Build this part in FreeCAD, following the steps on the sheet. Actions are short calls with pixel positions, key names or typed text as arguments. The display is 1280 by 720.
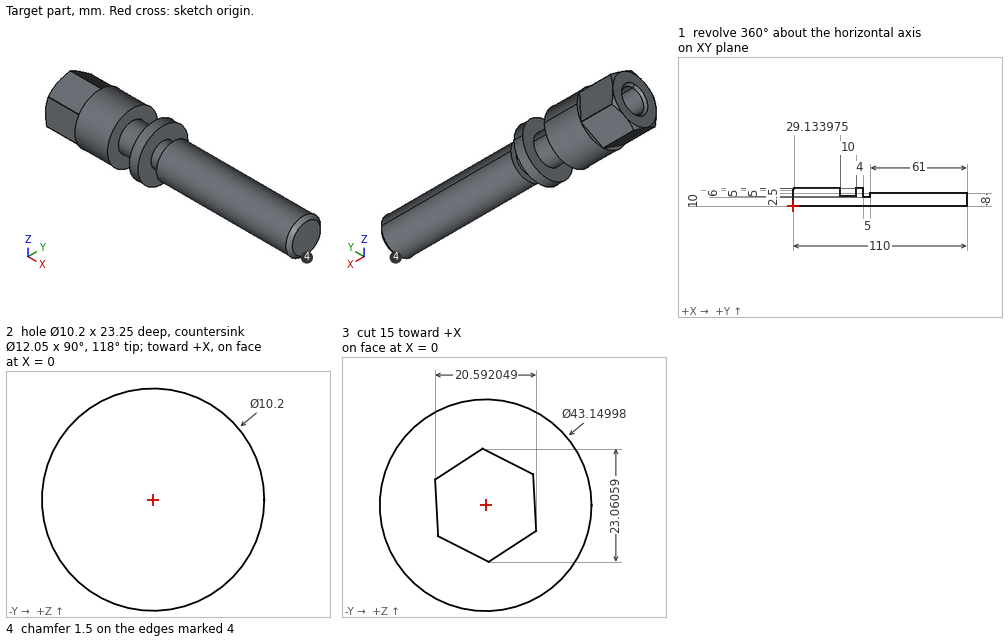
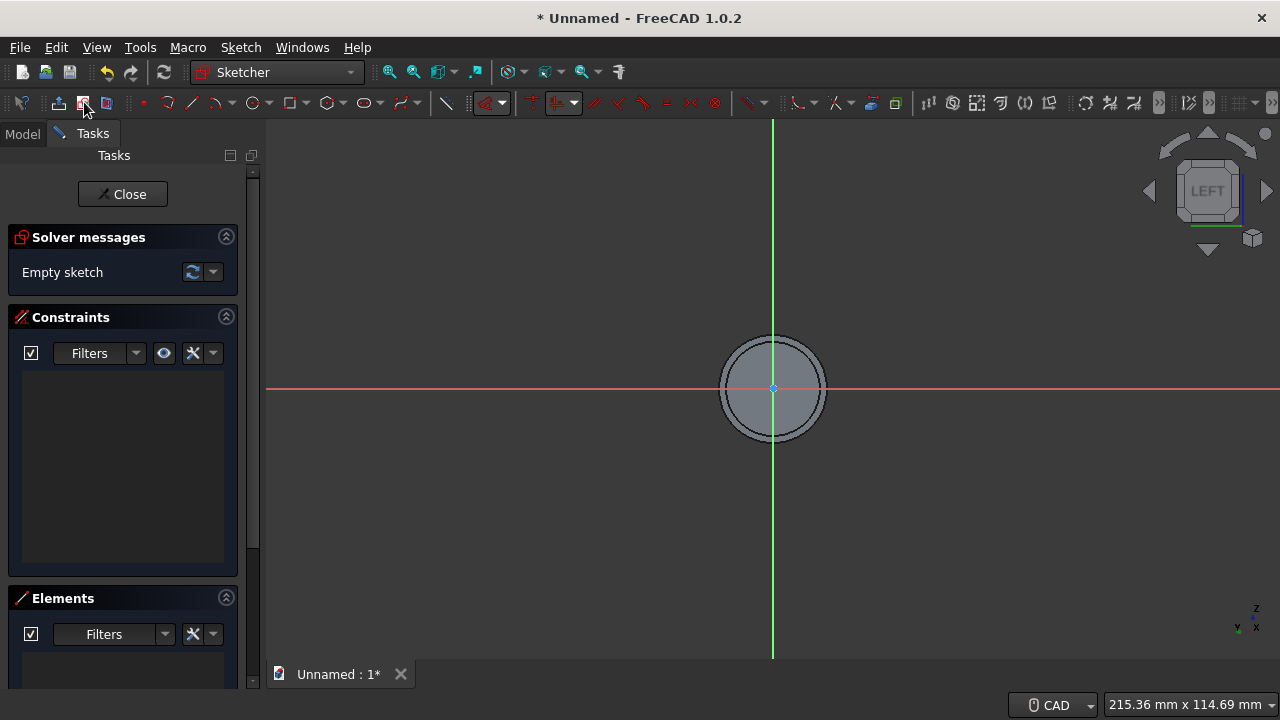
scroll(784, 389, up, 10)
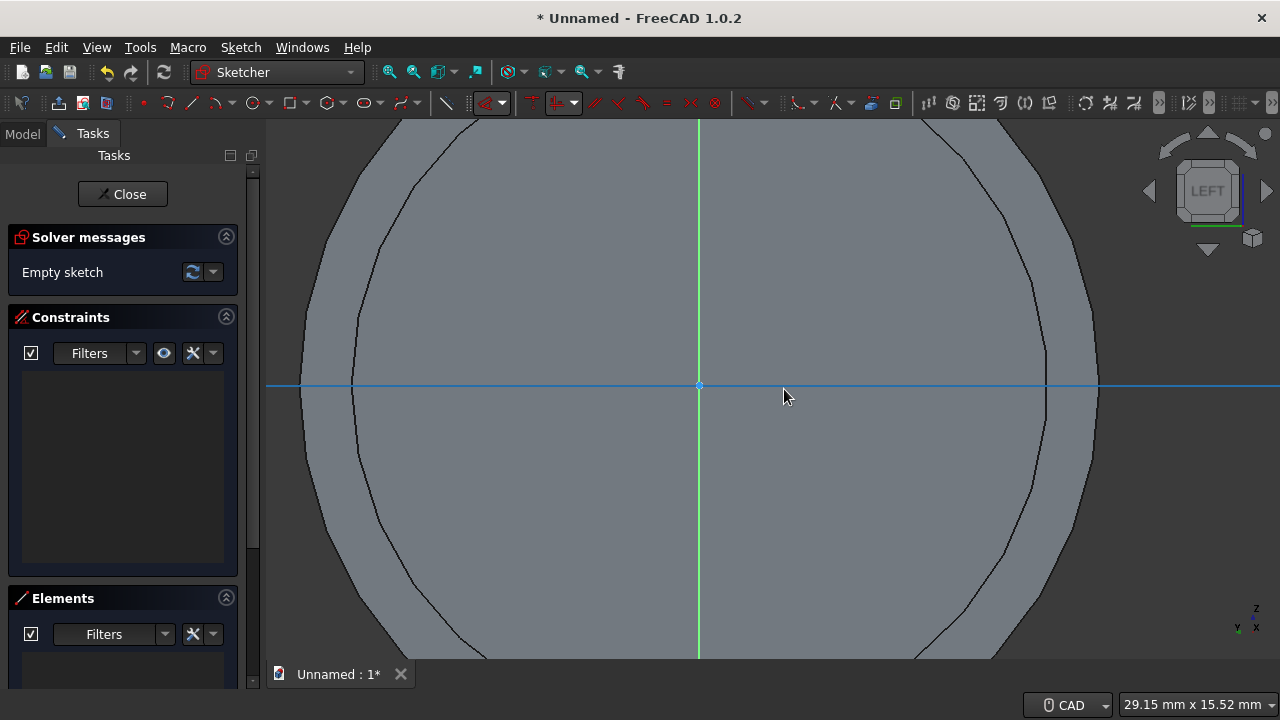
key(g)
key(c)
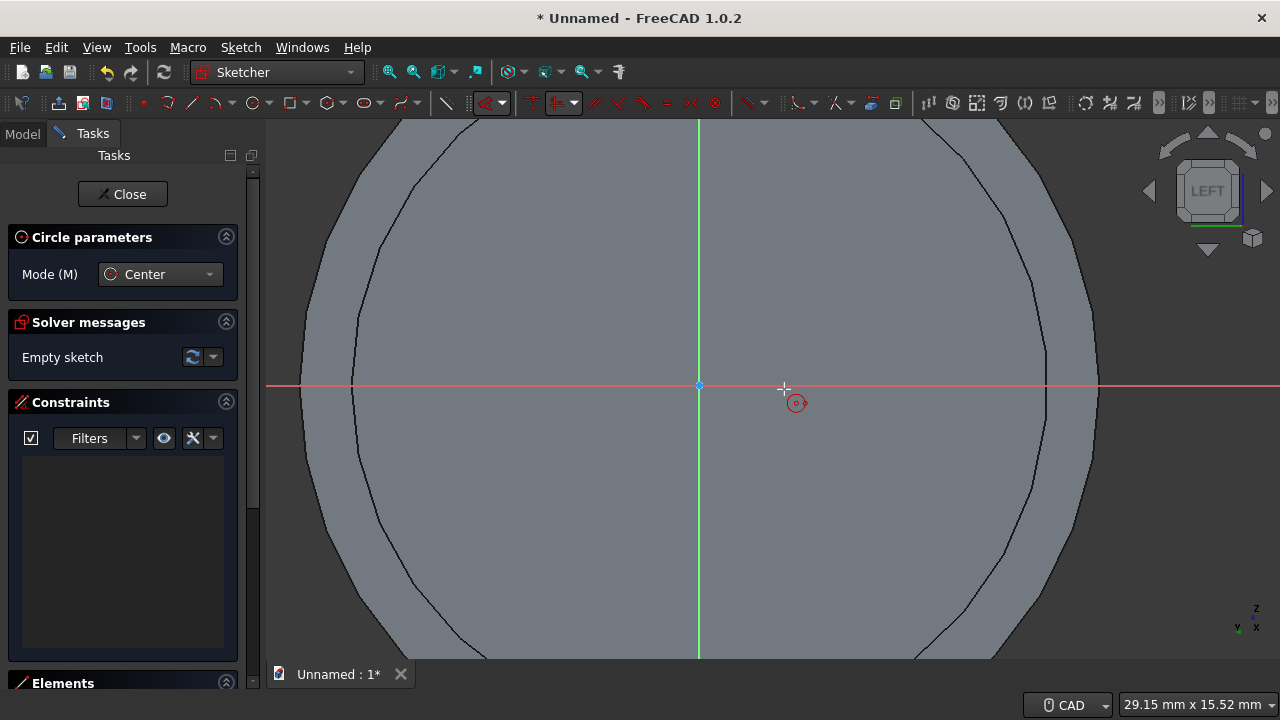
click(699, 386)
move(825, 260)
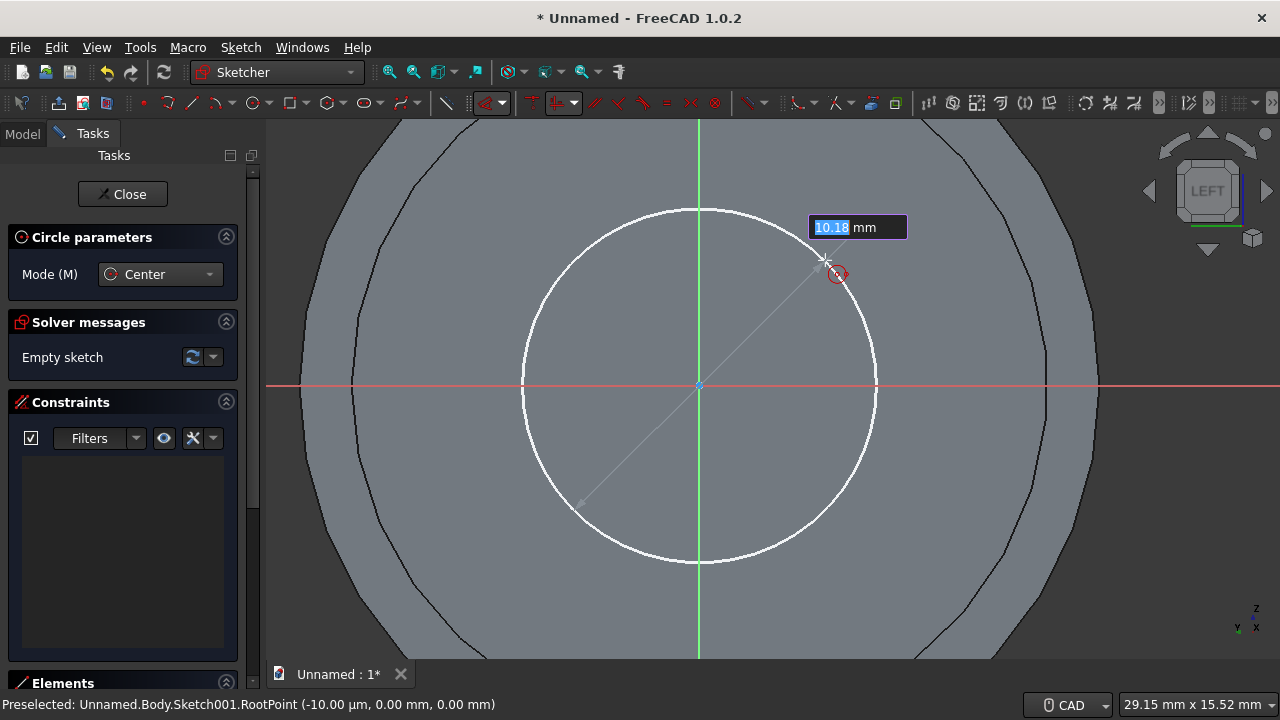
text(10.2)
key(Return)
key(Escape)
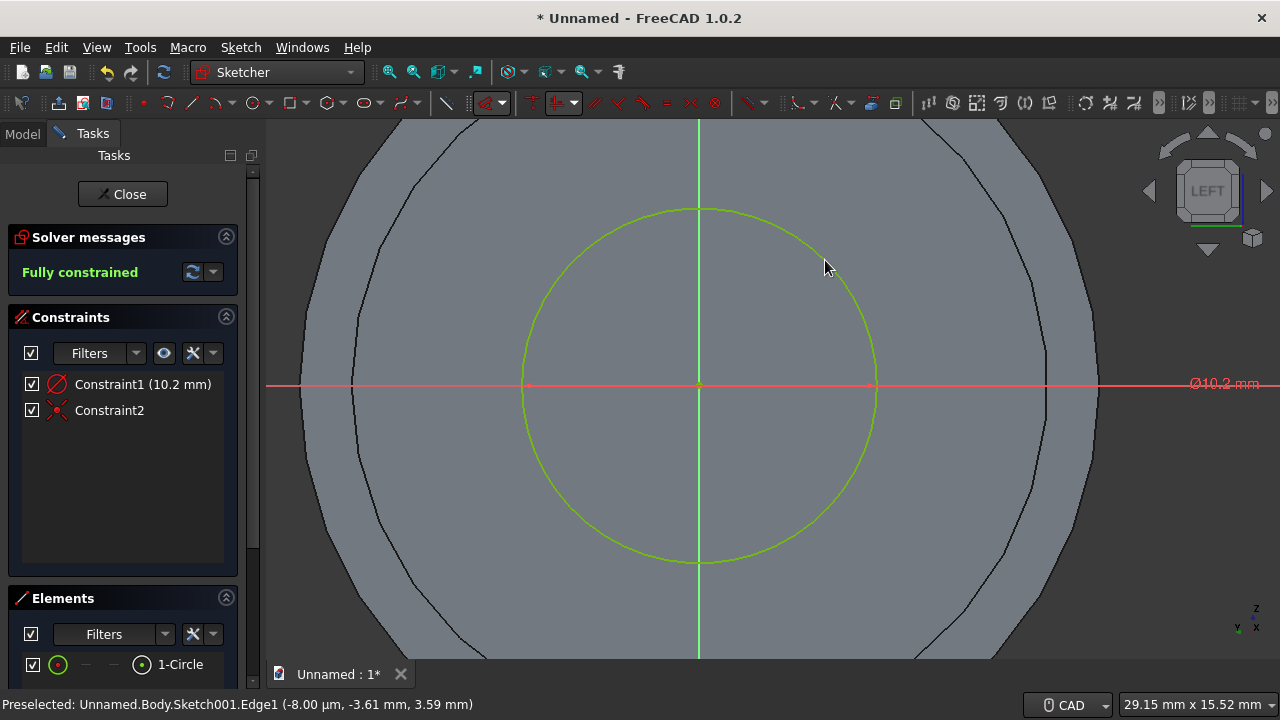
click(123, 194)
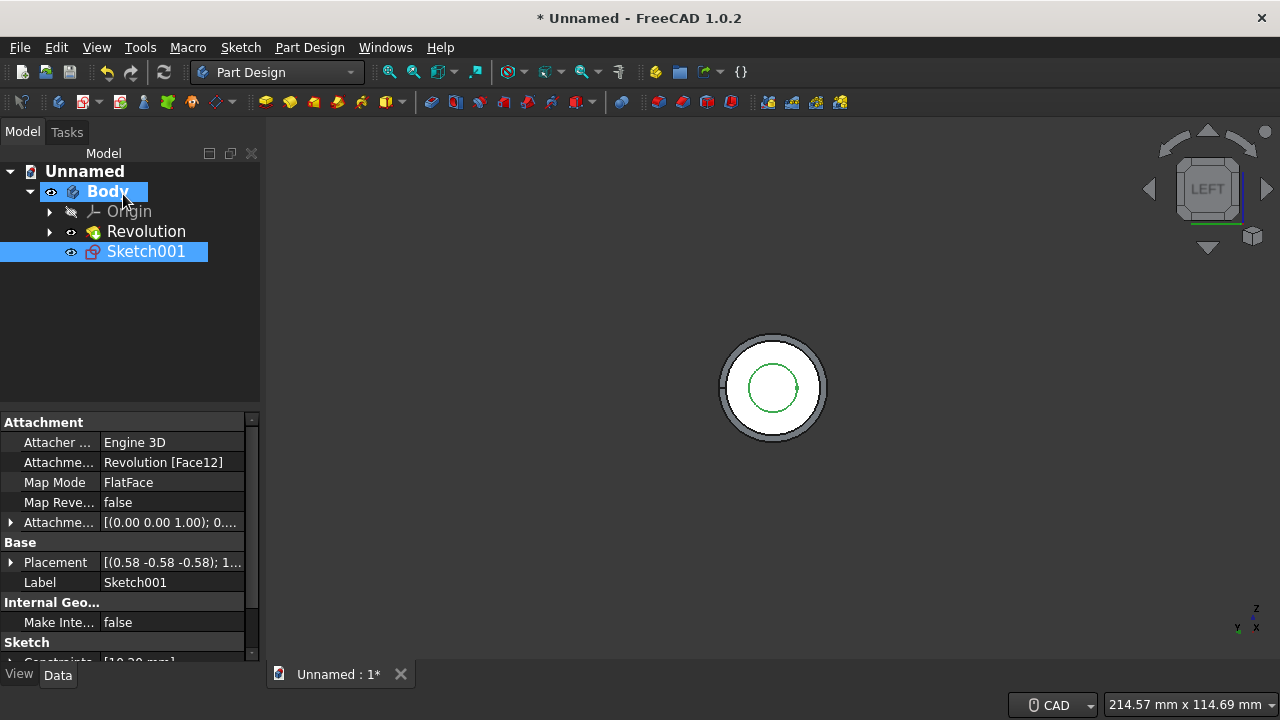
click(456, 102)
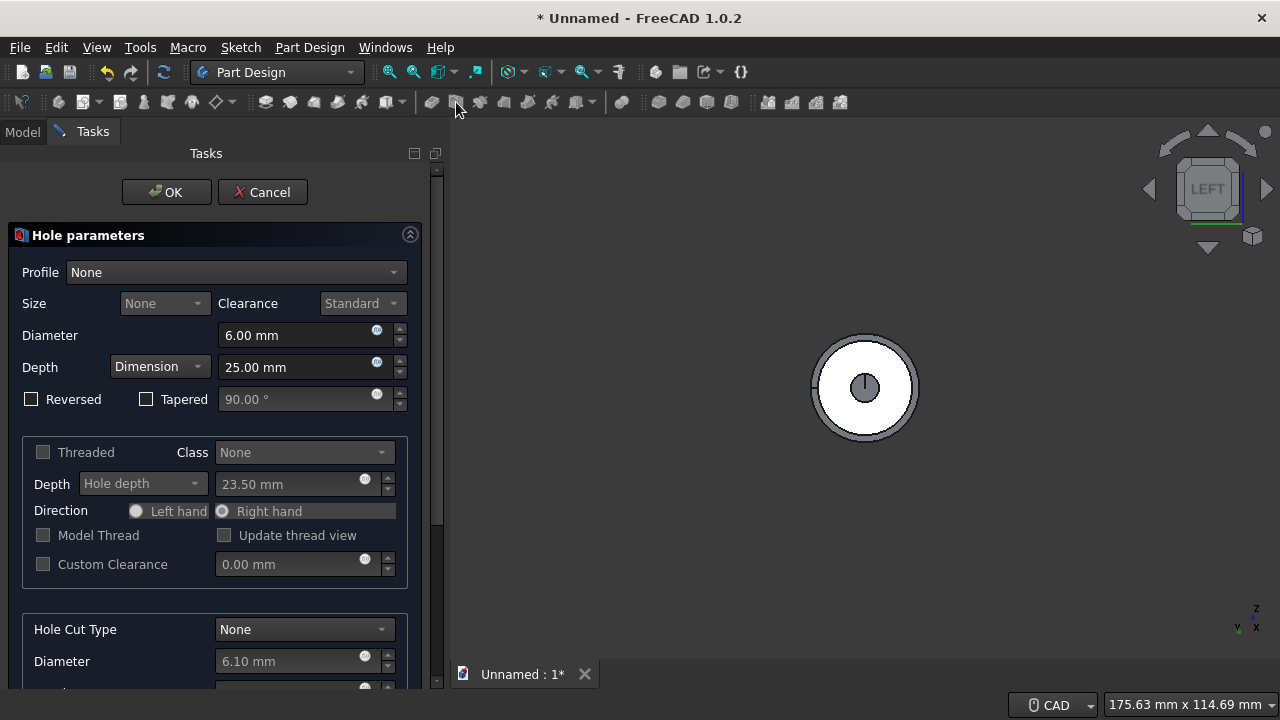
triple_click(305, 335)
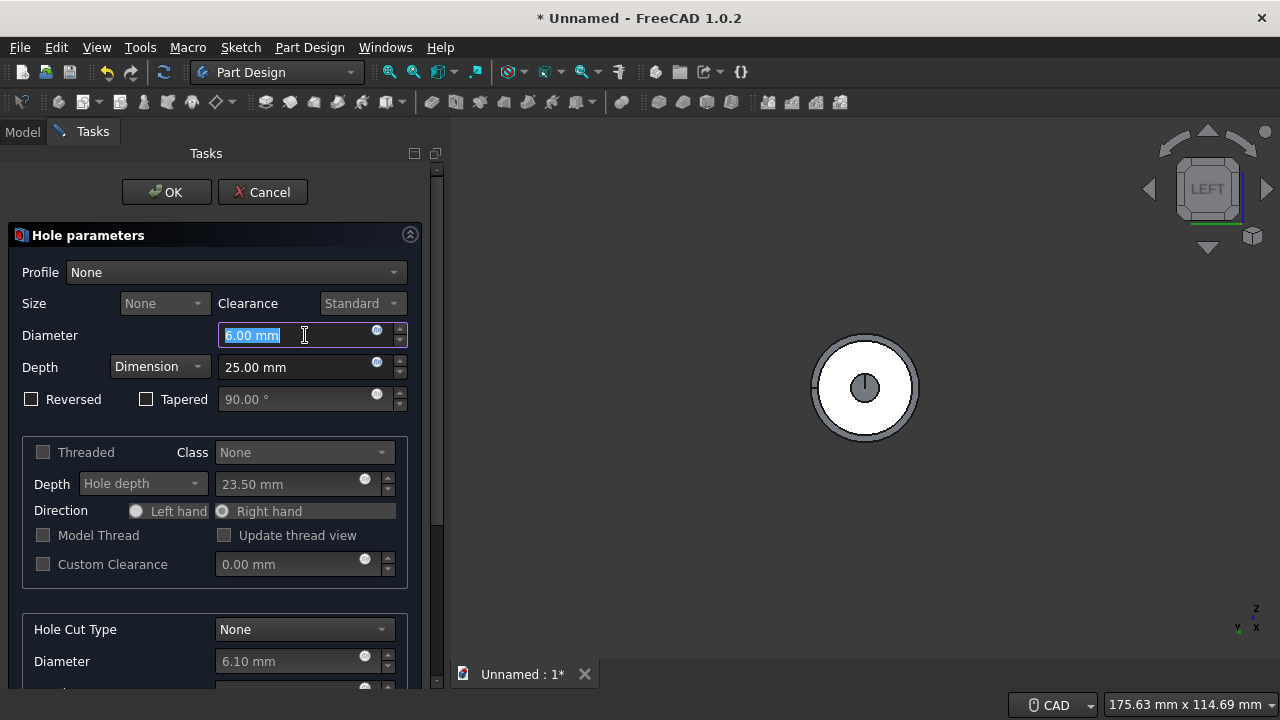
text(10.2)
key(Tab)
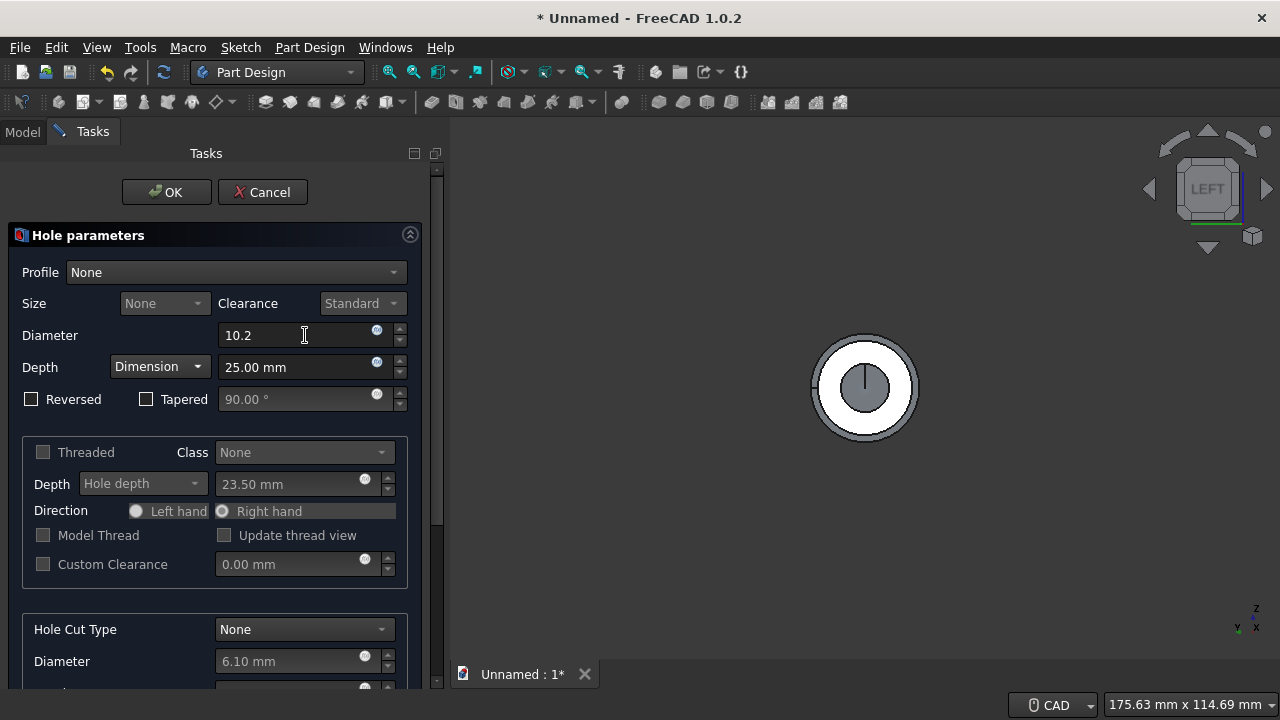
triple_click(305, 367)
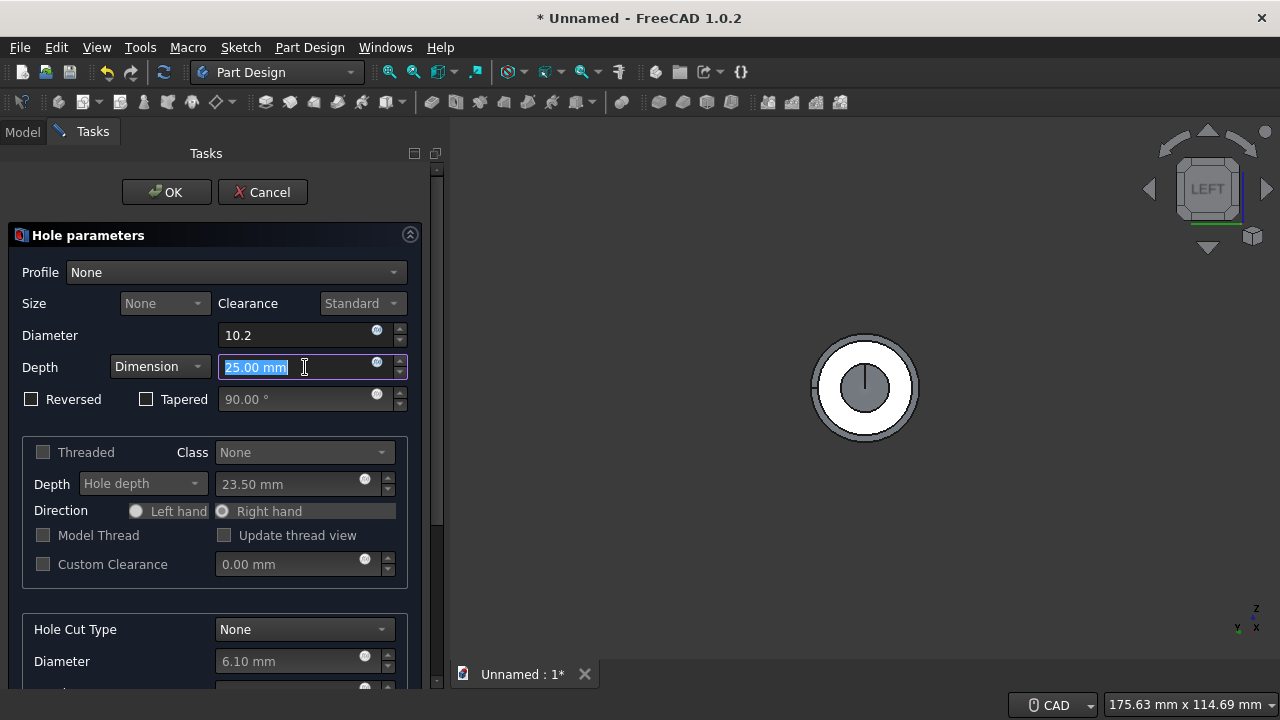
text(23.25)
key(Tab)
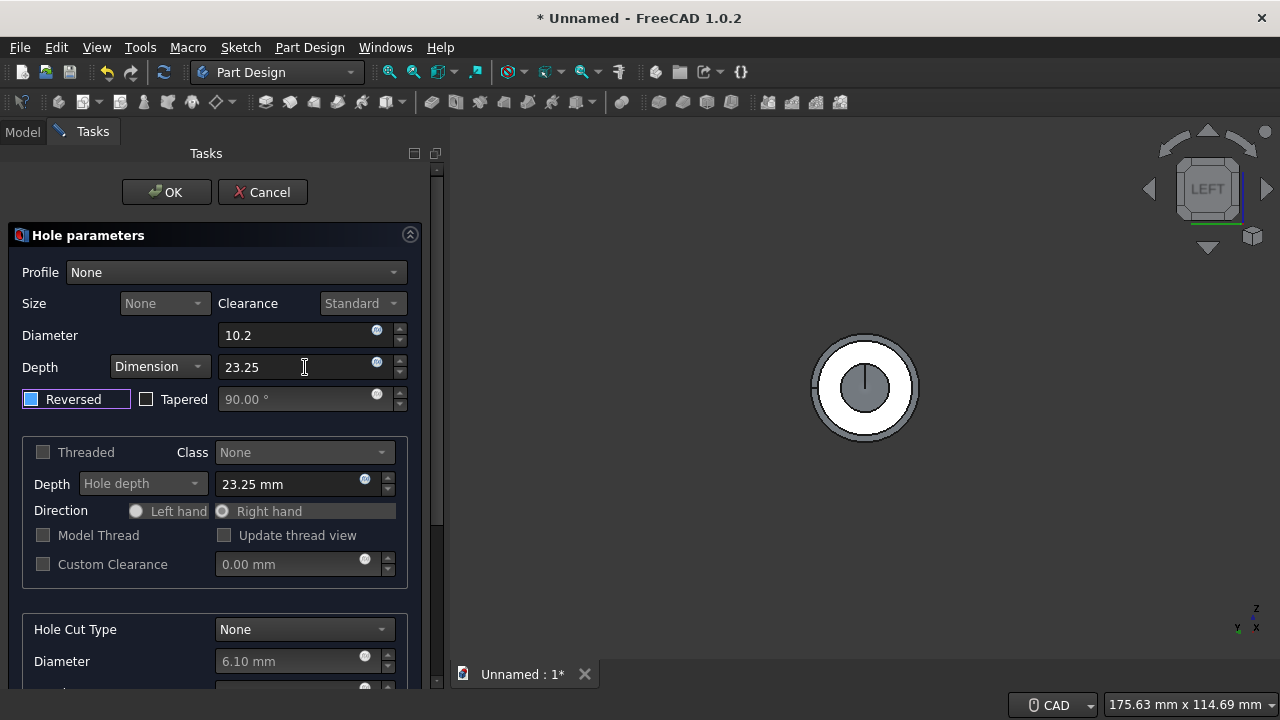
click(306, 630)